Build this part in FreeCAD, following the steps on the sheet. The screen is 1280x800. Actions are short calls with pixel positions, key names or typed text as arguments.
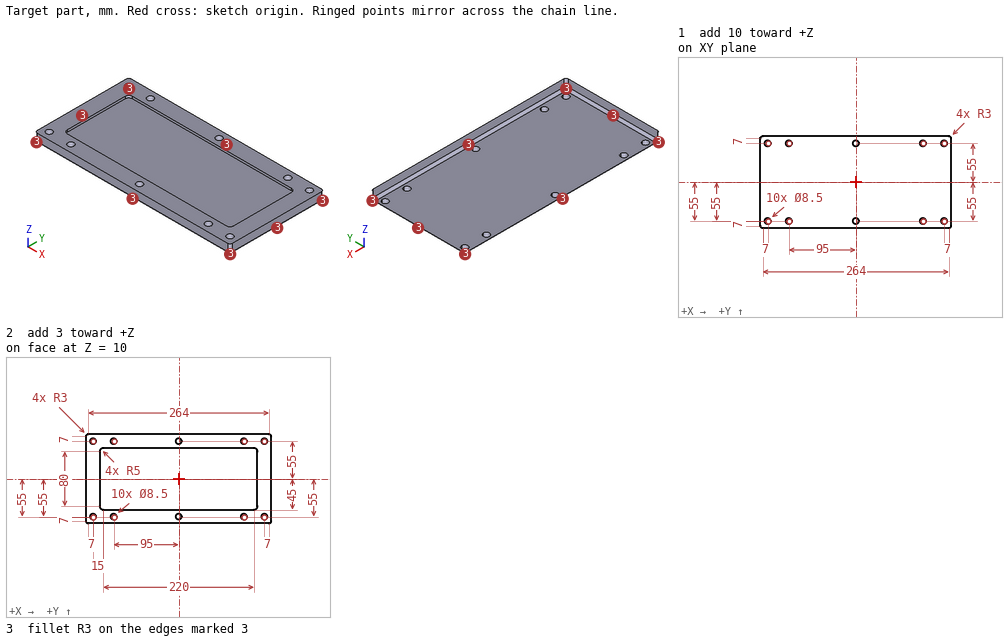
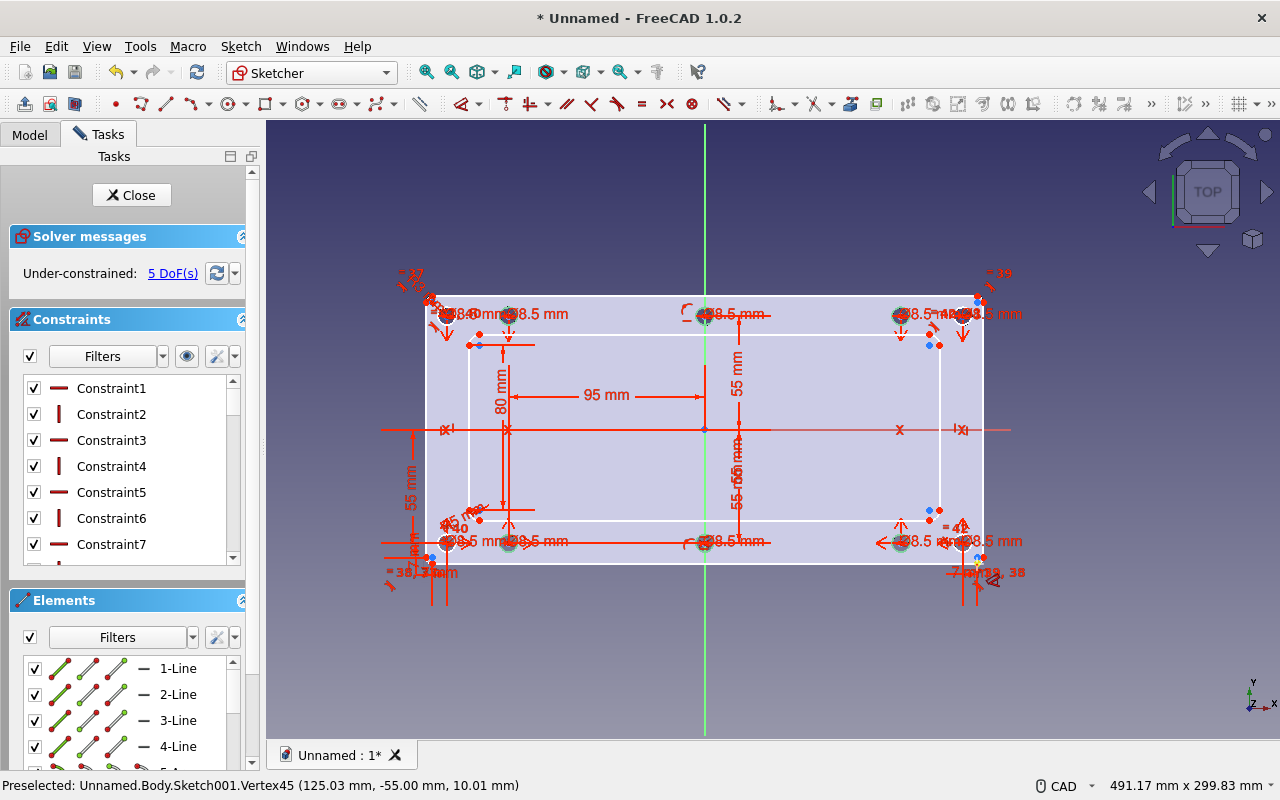
scroll(426, 303, up, 6)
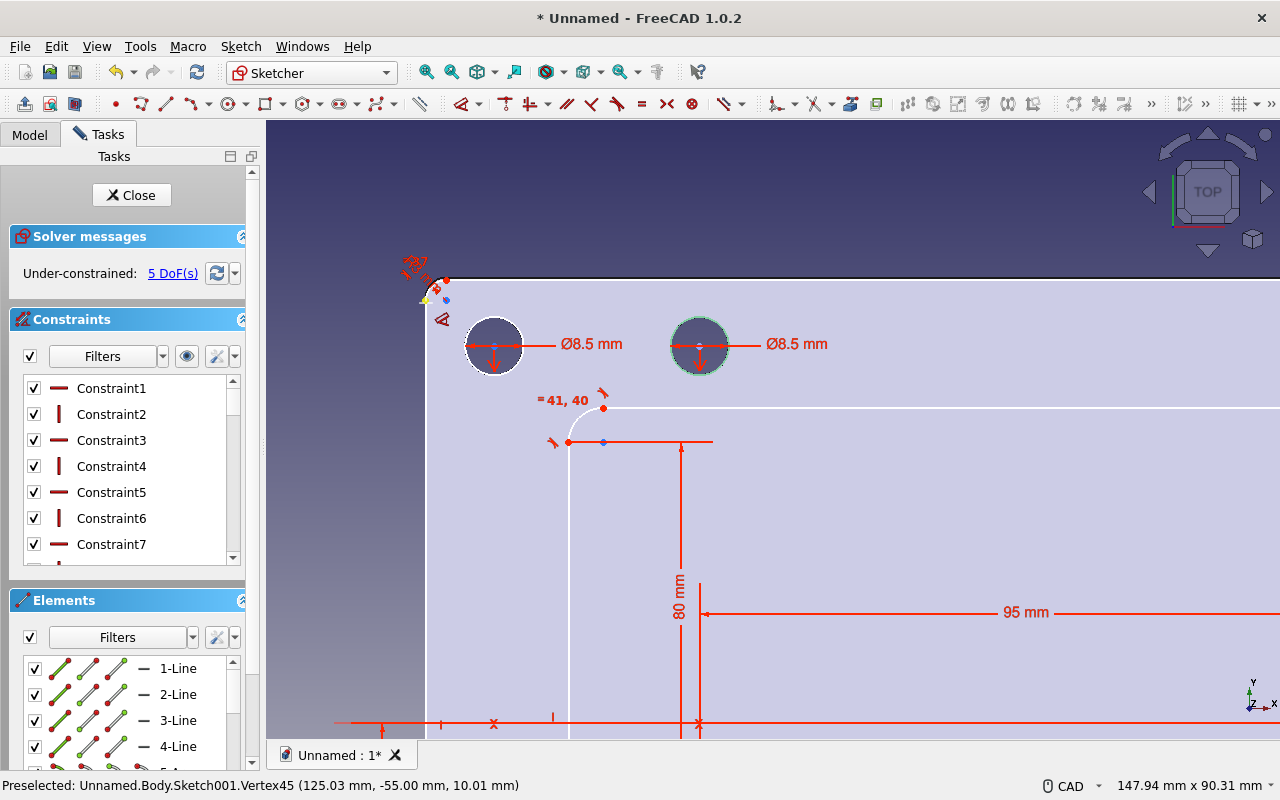
click(426, 301)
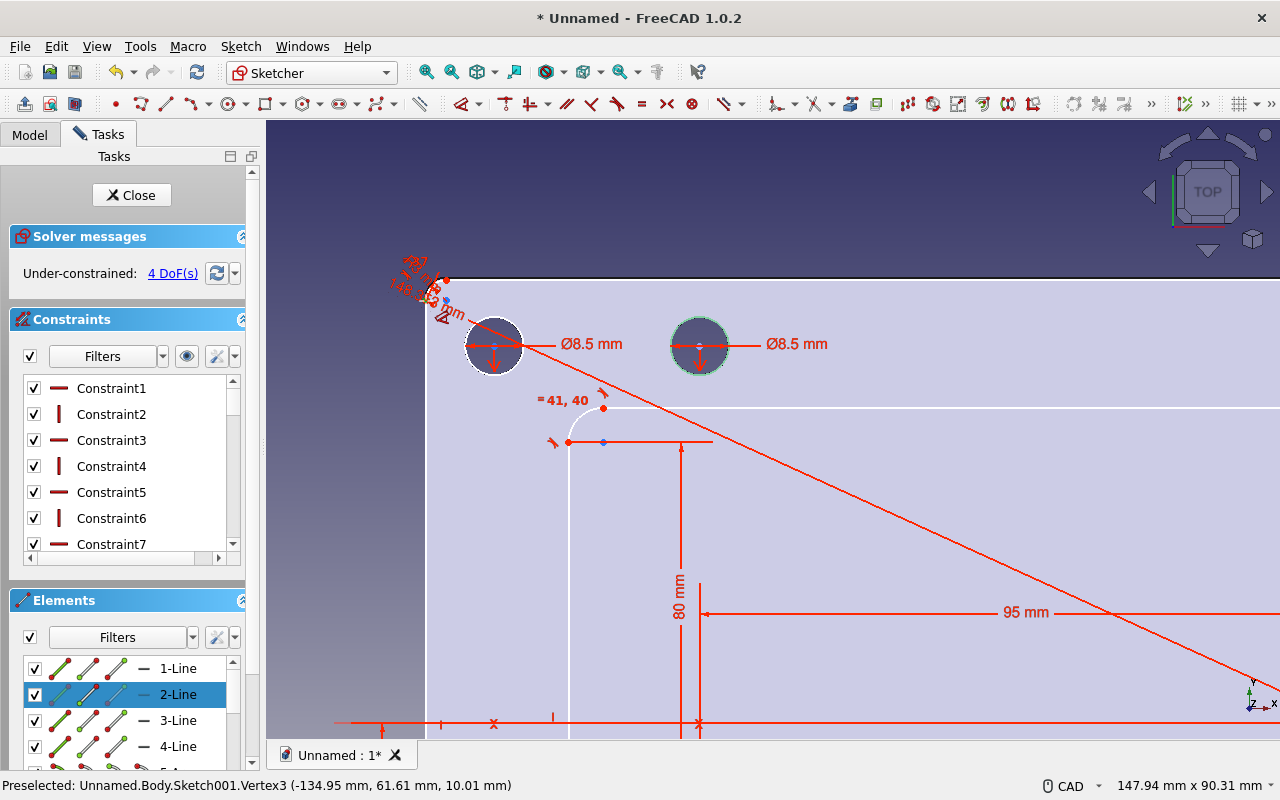
click(494, 346)
click(392, 323)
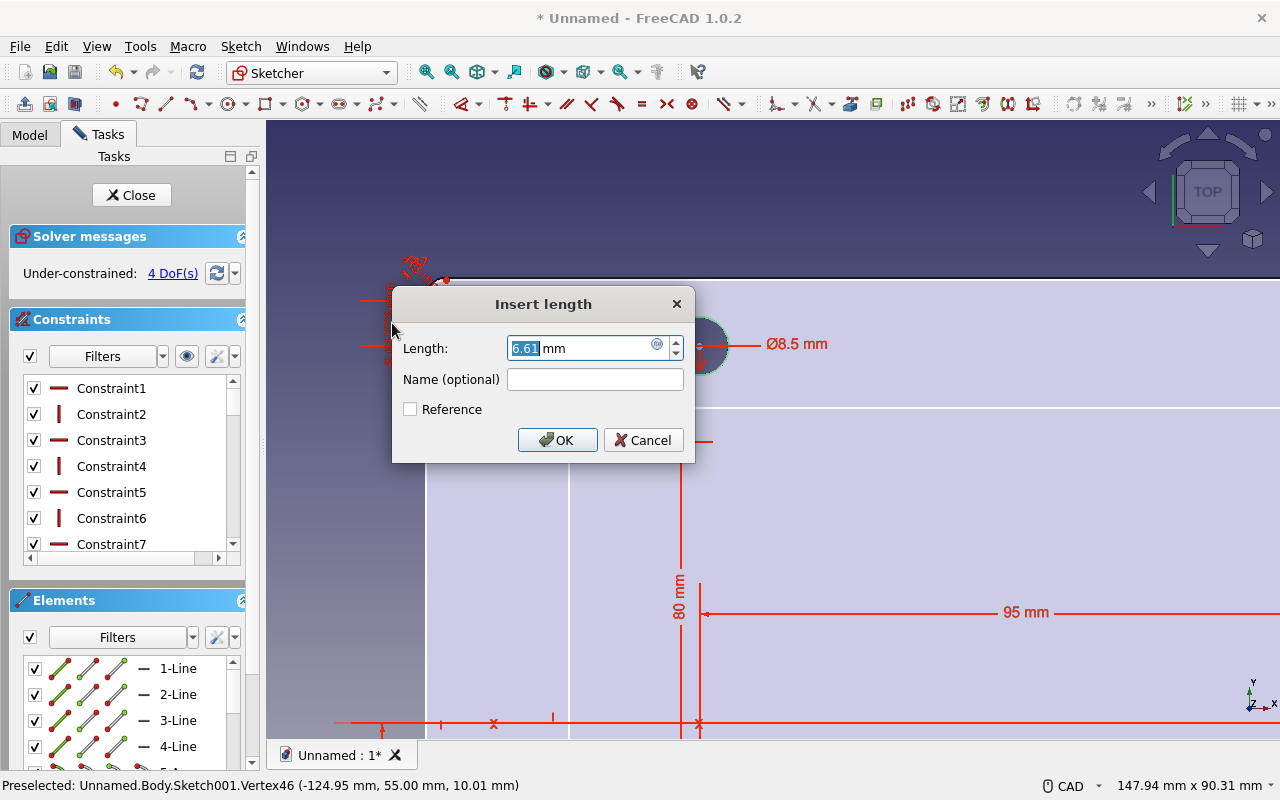
text(7)
key(Return)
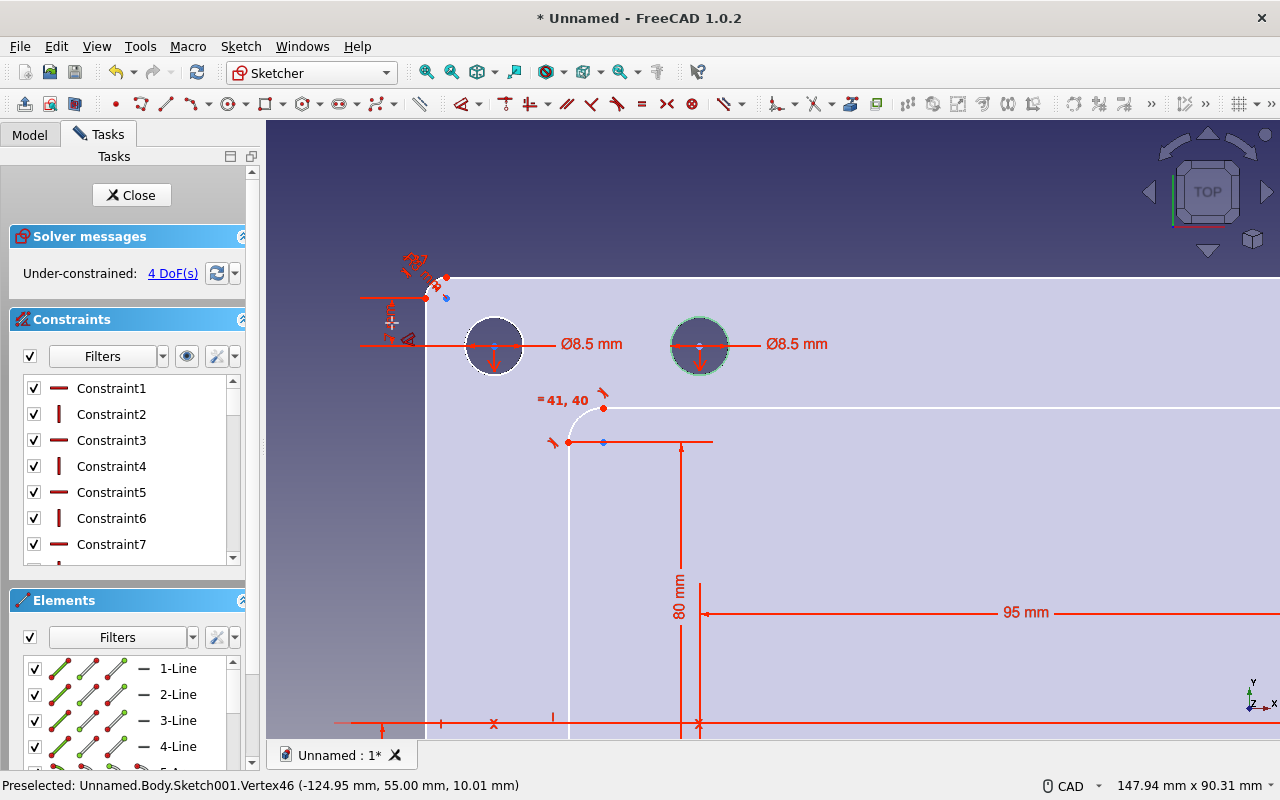
click(989, 278)
click(781, 244)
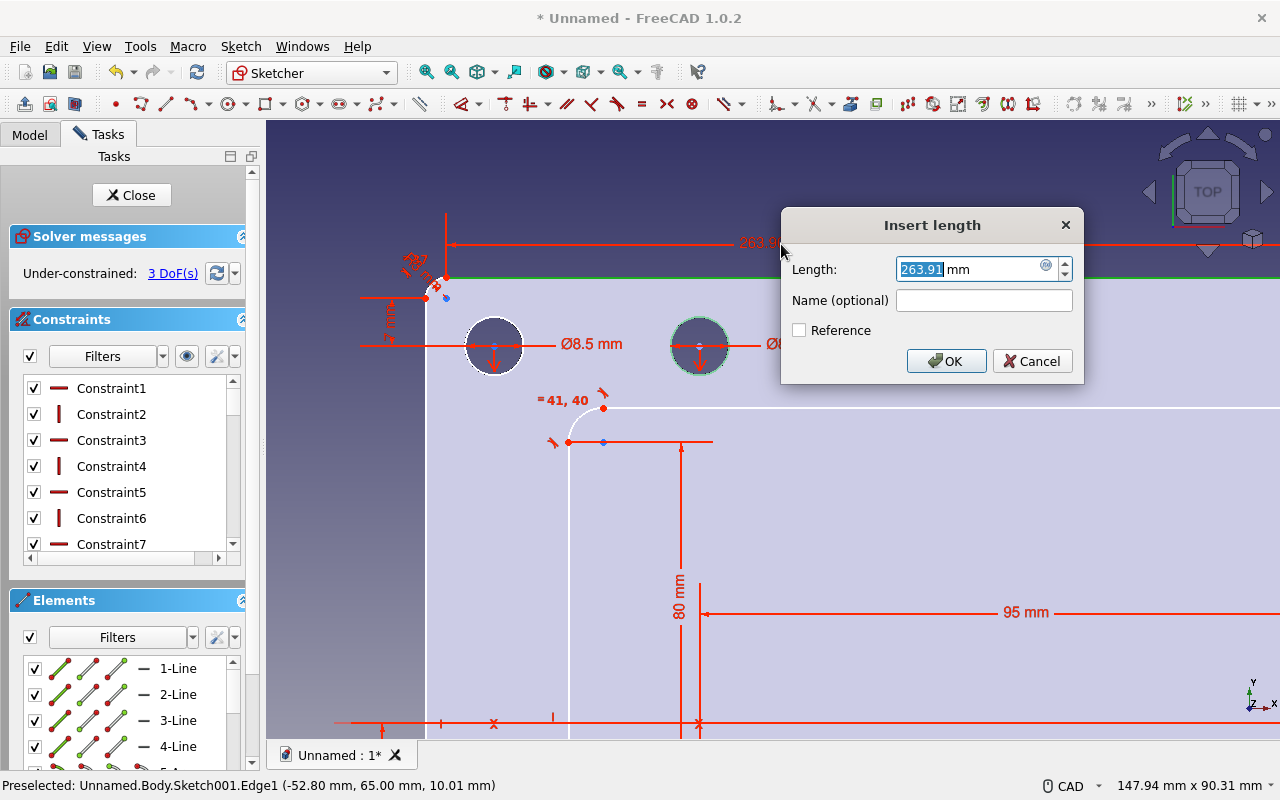
text(264)
key(Return)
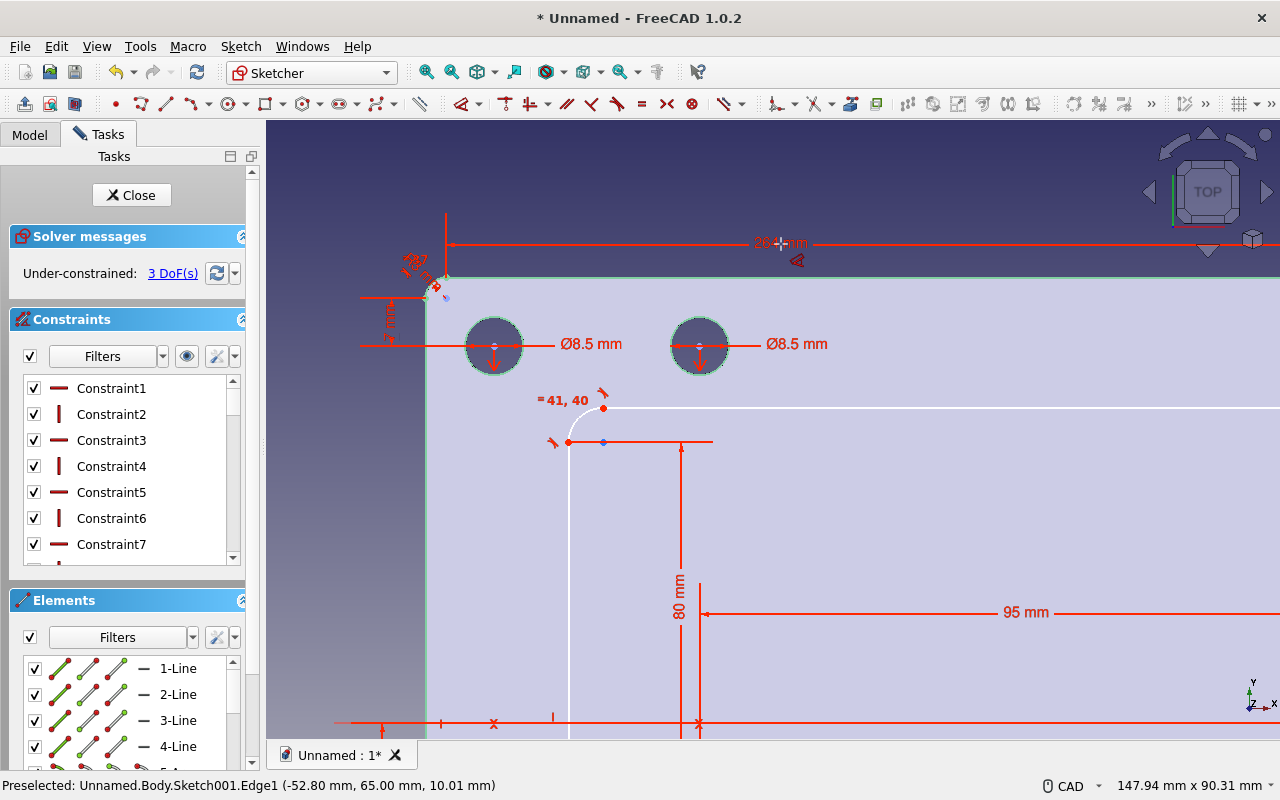
scroll(426, 303, down, 6)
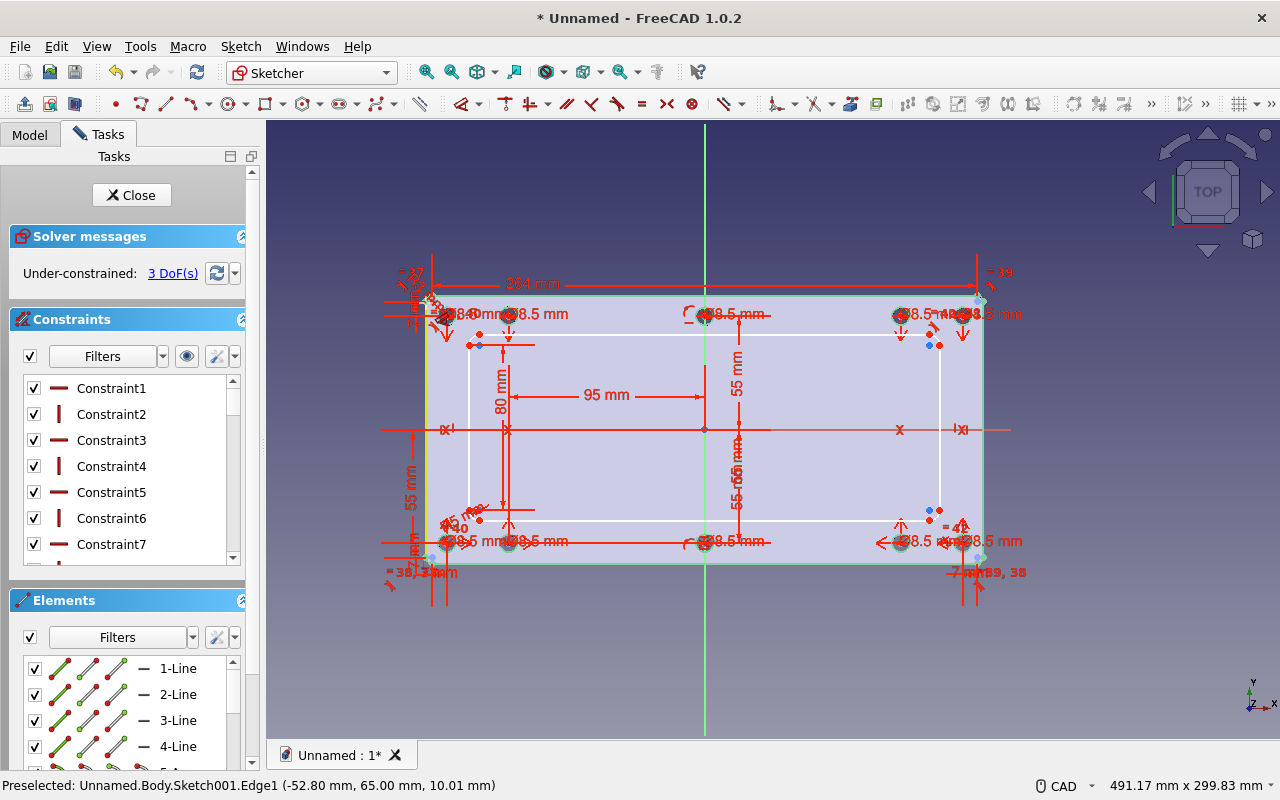
click(794, 521)
click(601, 487)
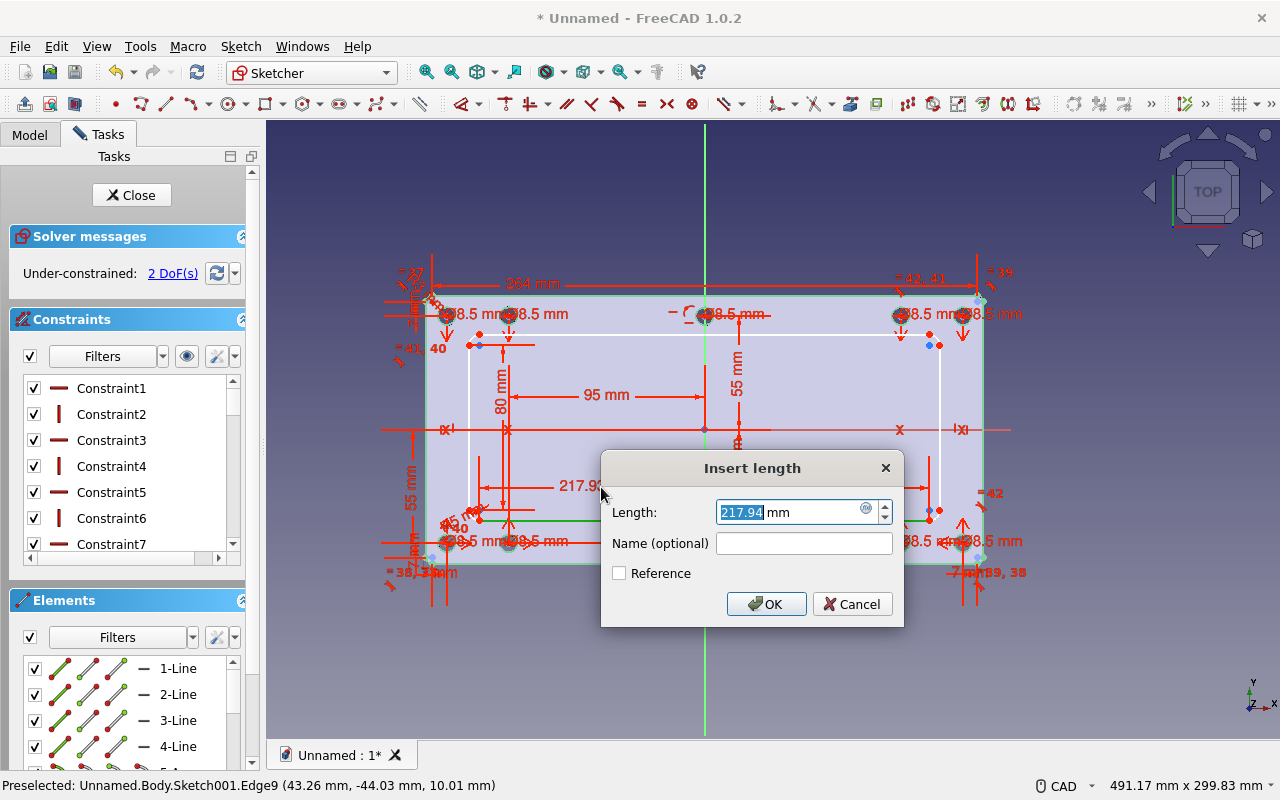
text(220)
key(Return)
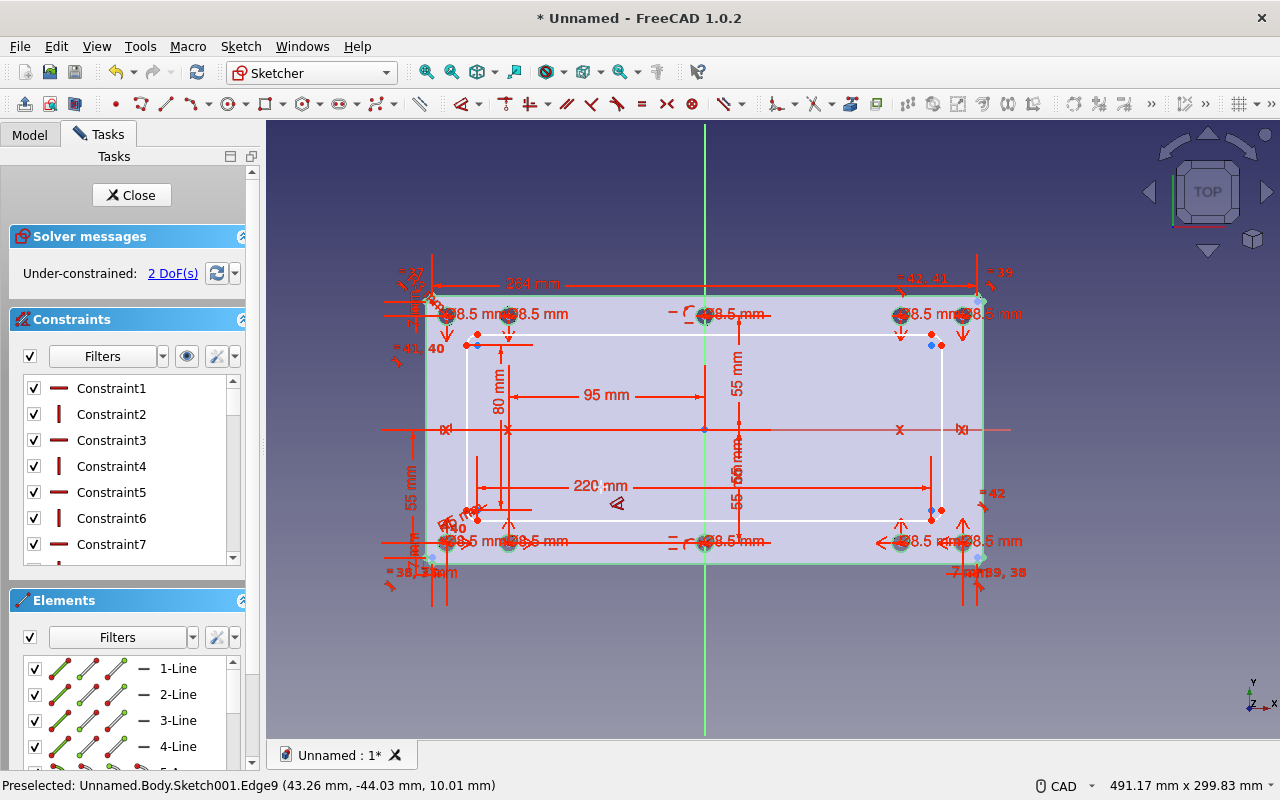
click(931, 521)
click(965, 475)